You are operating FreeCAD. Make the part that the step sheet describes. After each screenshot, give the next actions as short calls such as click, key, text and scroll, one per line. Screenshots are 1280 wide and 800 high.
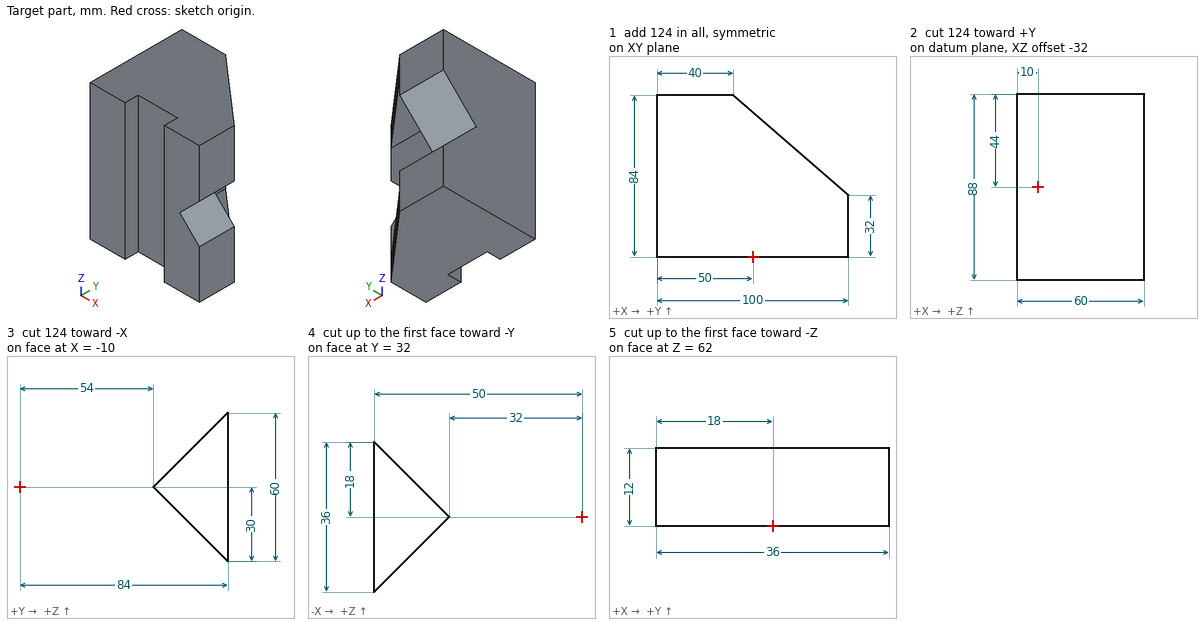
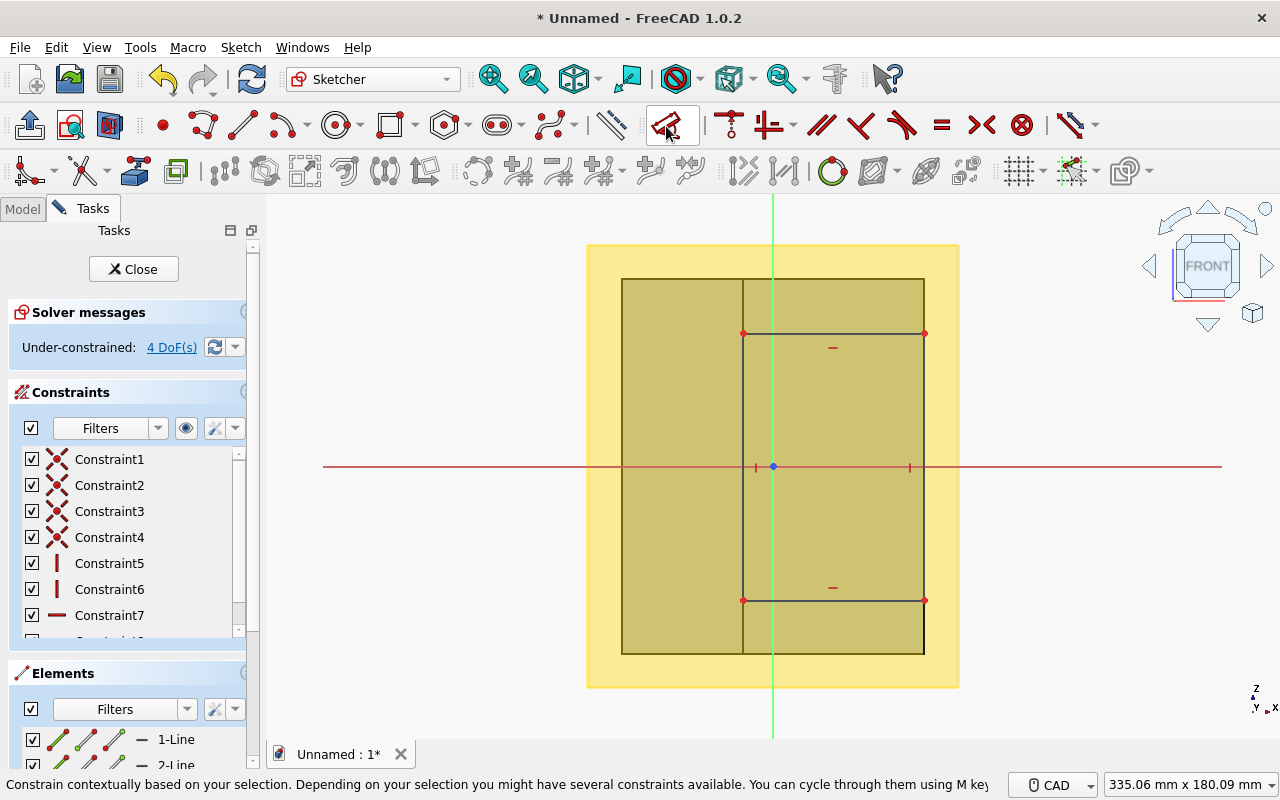
click(743, 414)
click(709, 406)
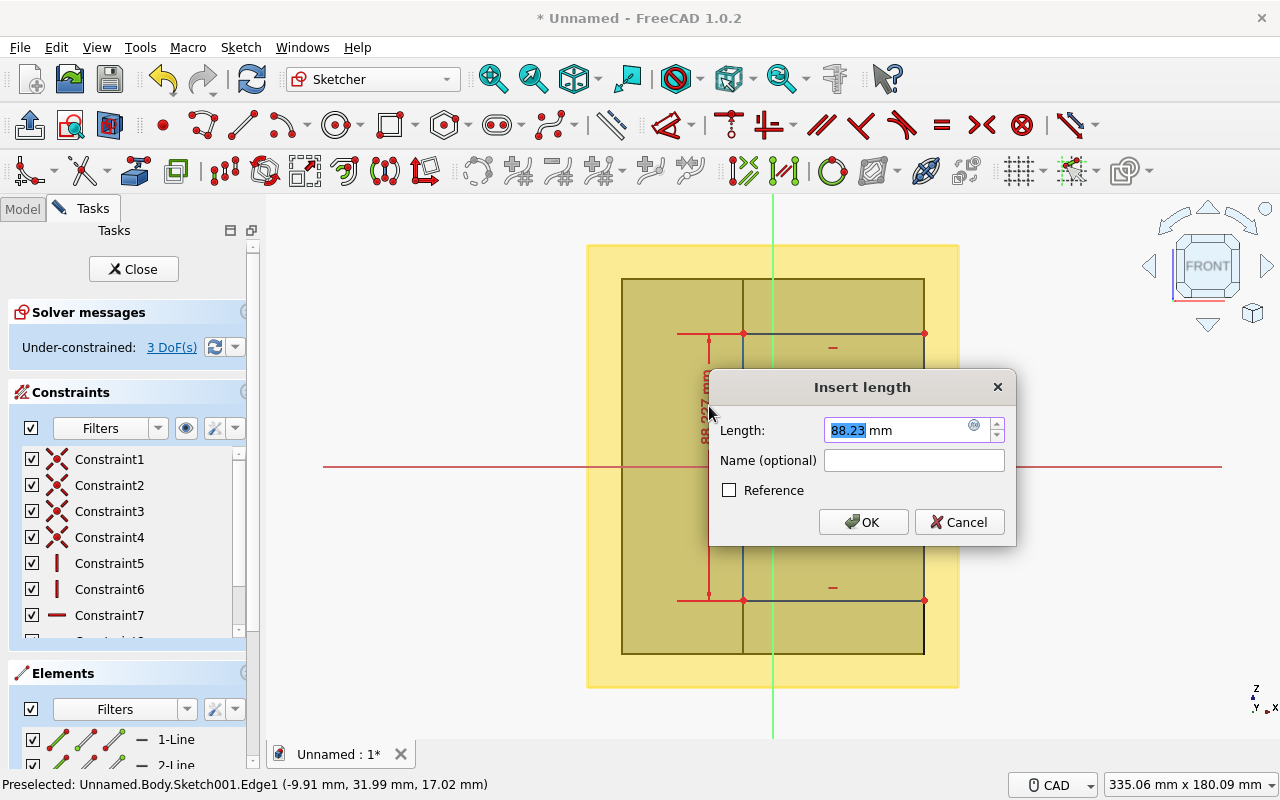
text(88)
key(Return)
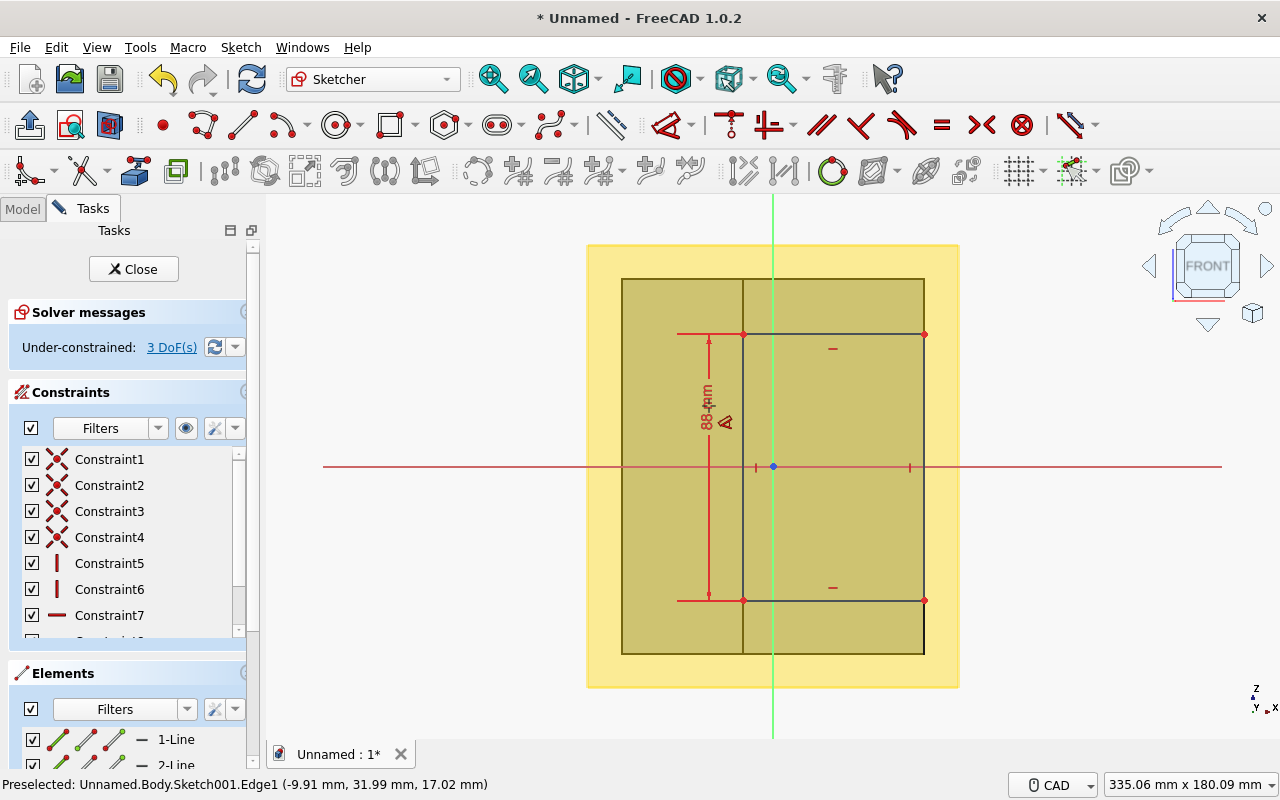
click(797, 601)
click(833, 635)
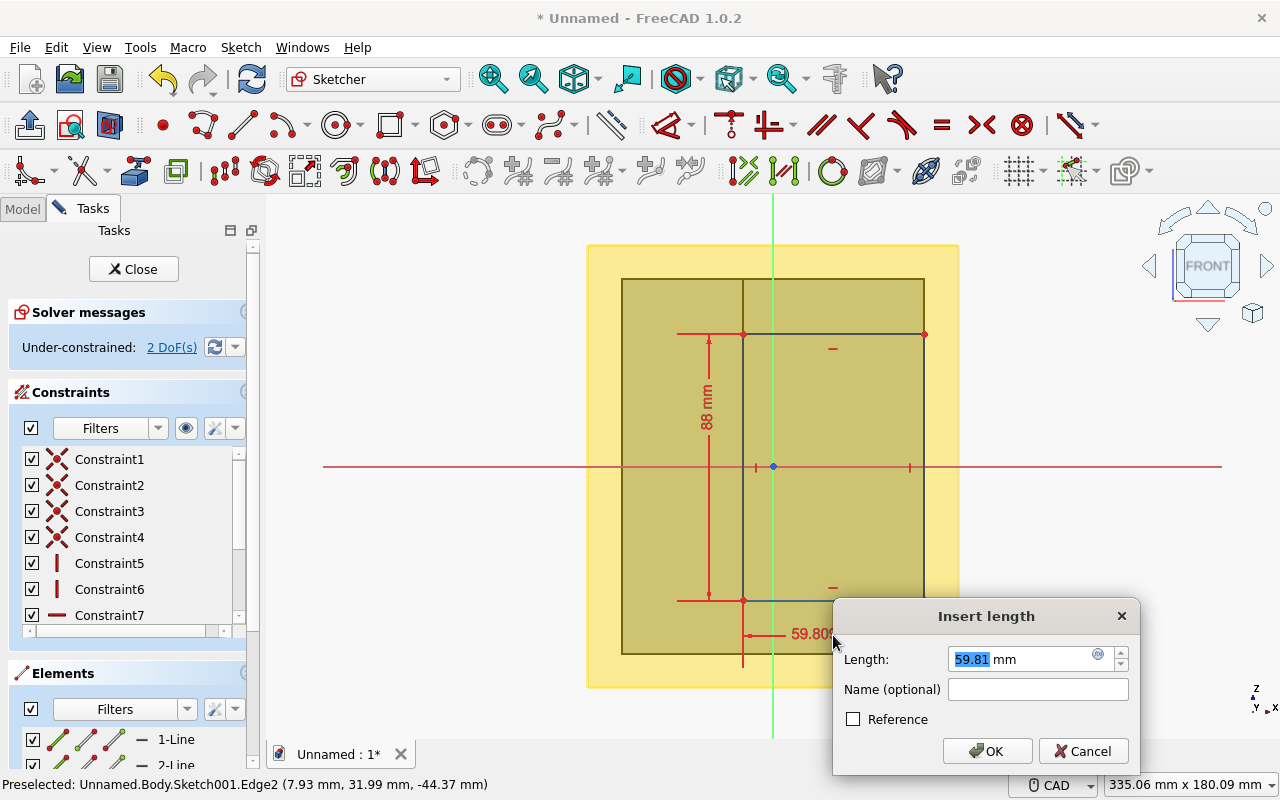
text(60)
key(Return)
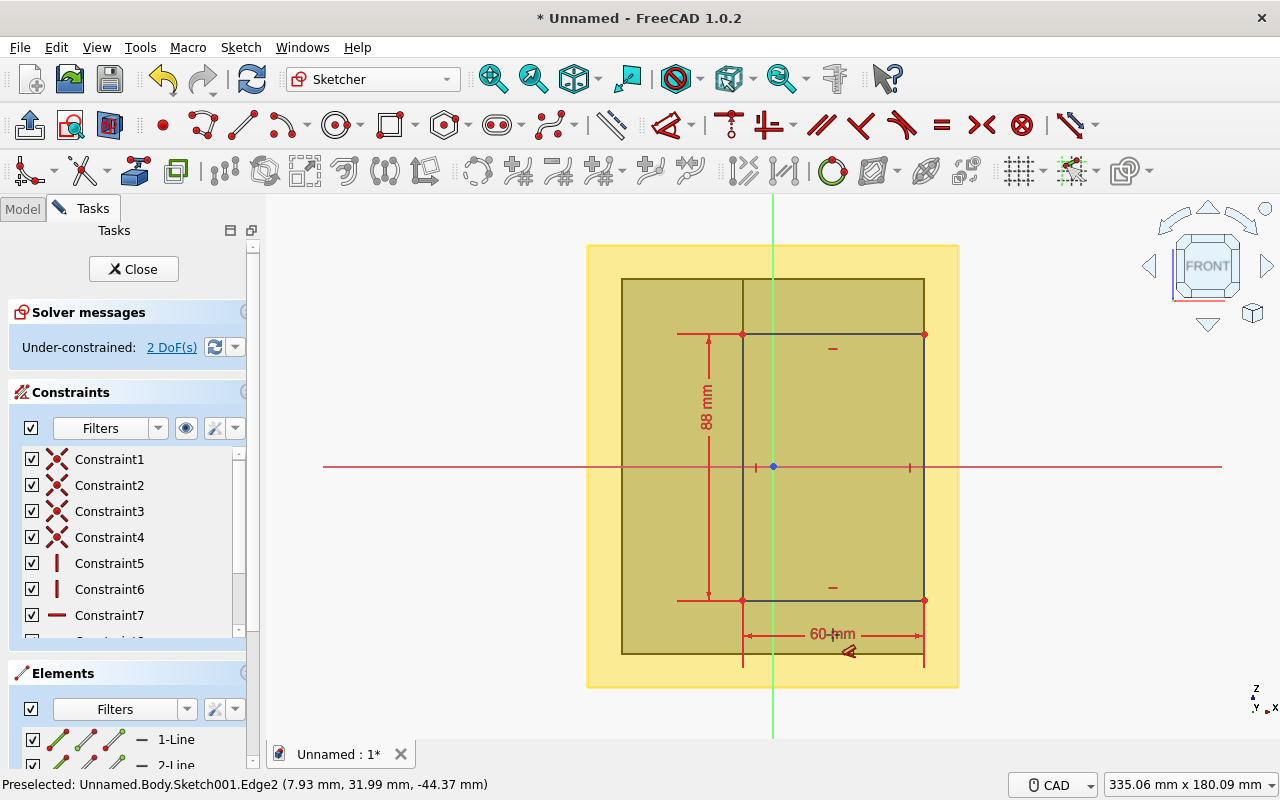
scroll(743, 334, up, 2)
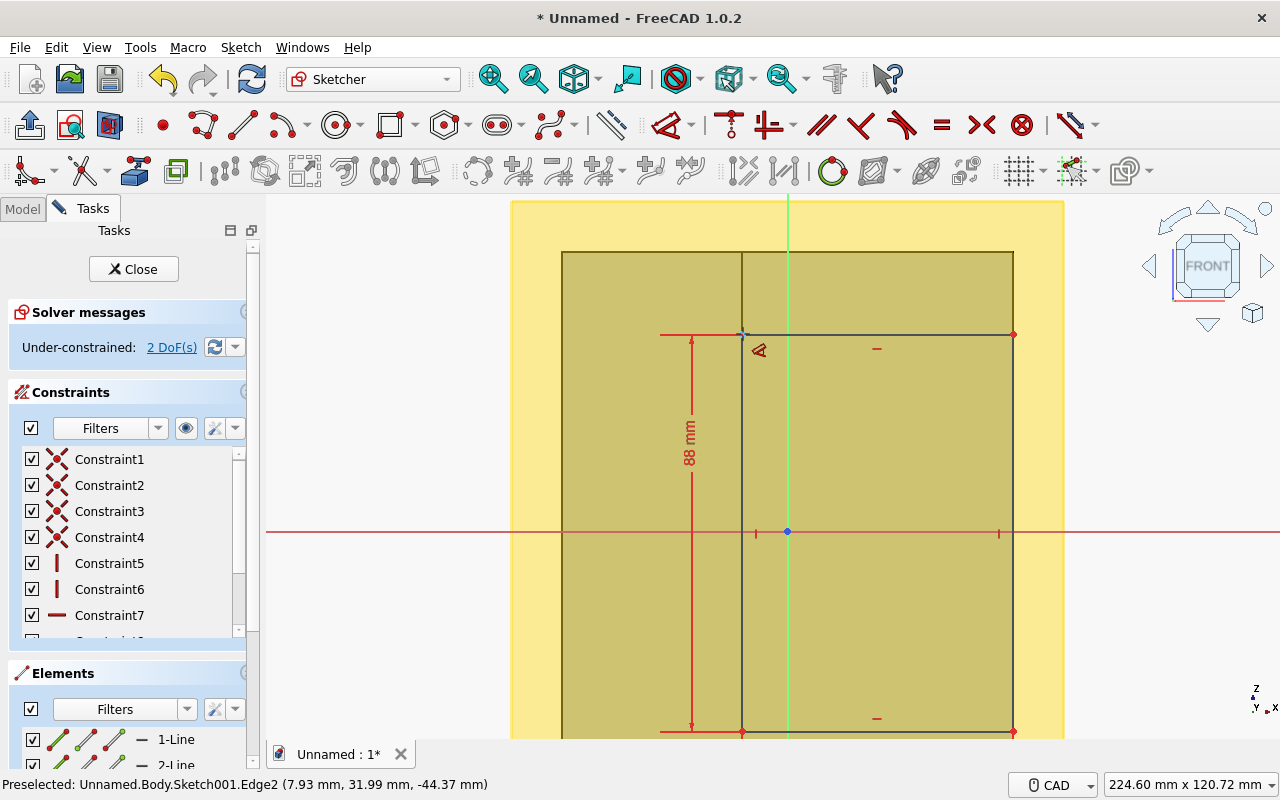
click(742, 335)
click(765, 301)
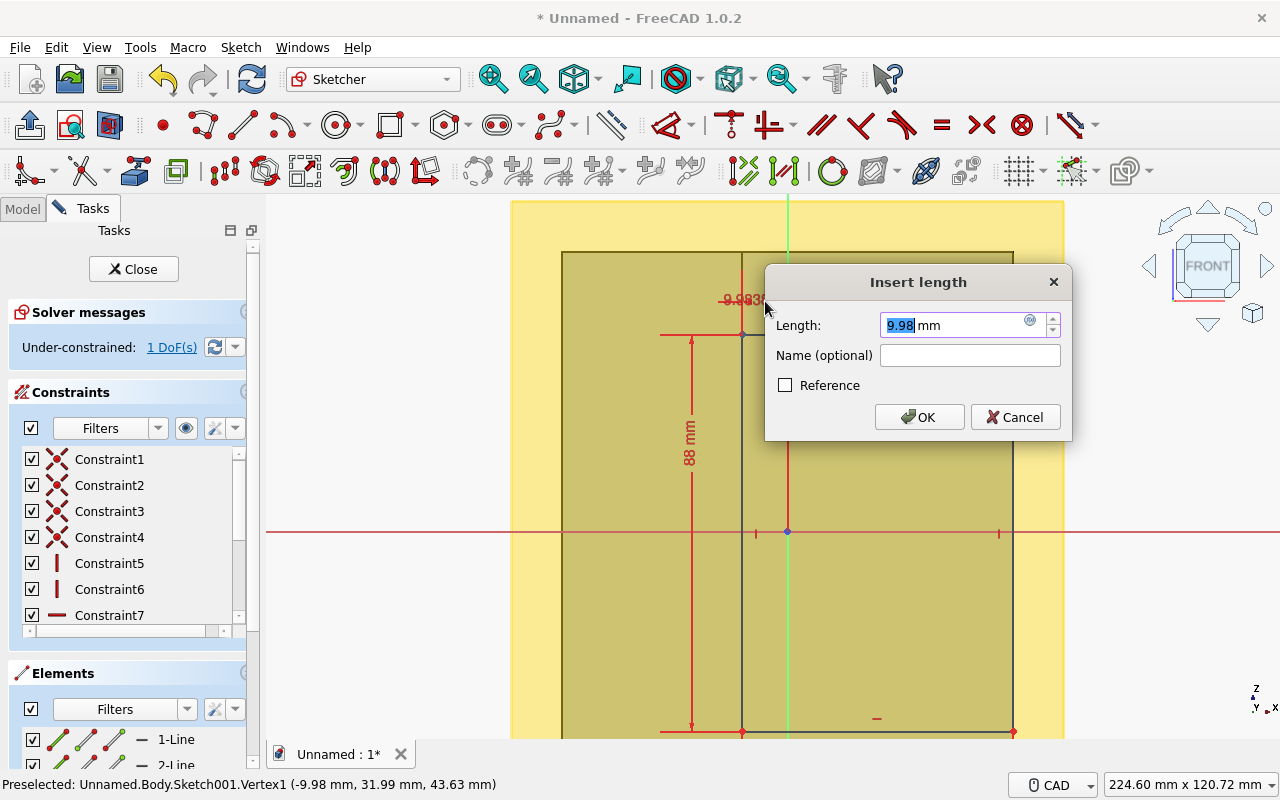
text(10)
key(Return)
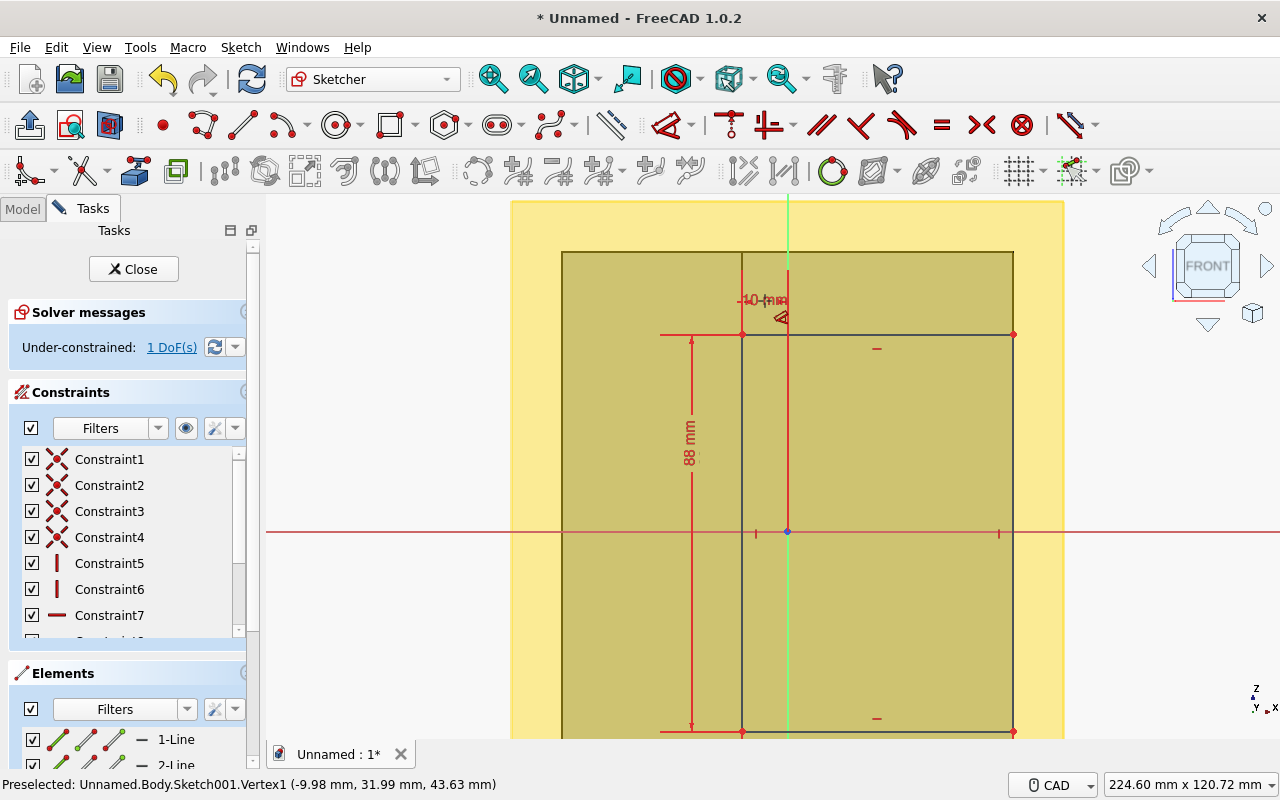
click(742, 335)
click(708, 388)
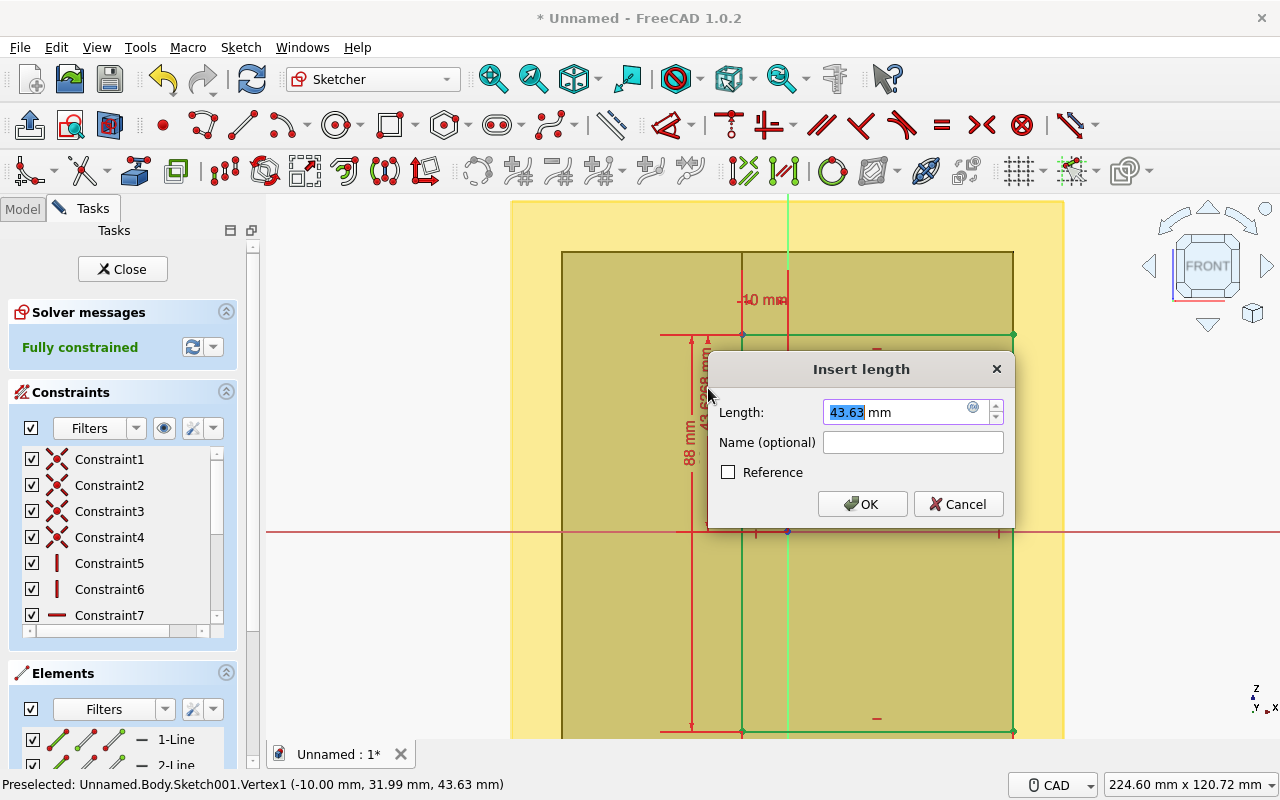
text(44)
key(Return)
key(Escape)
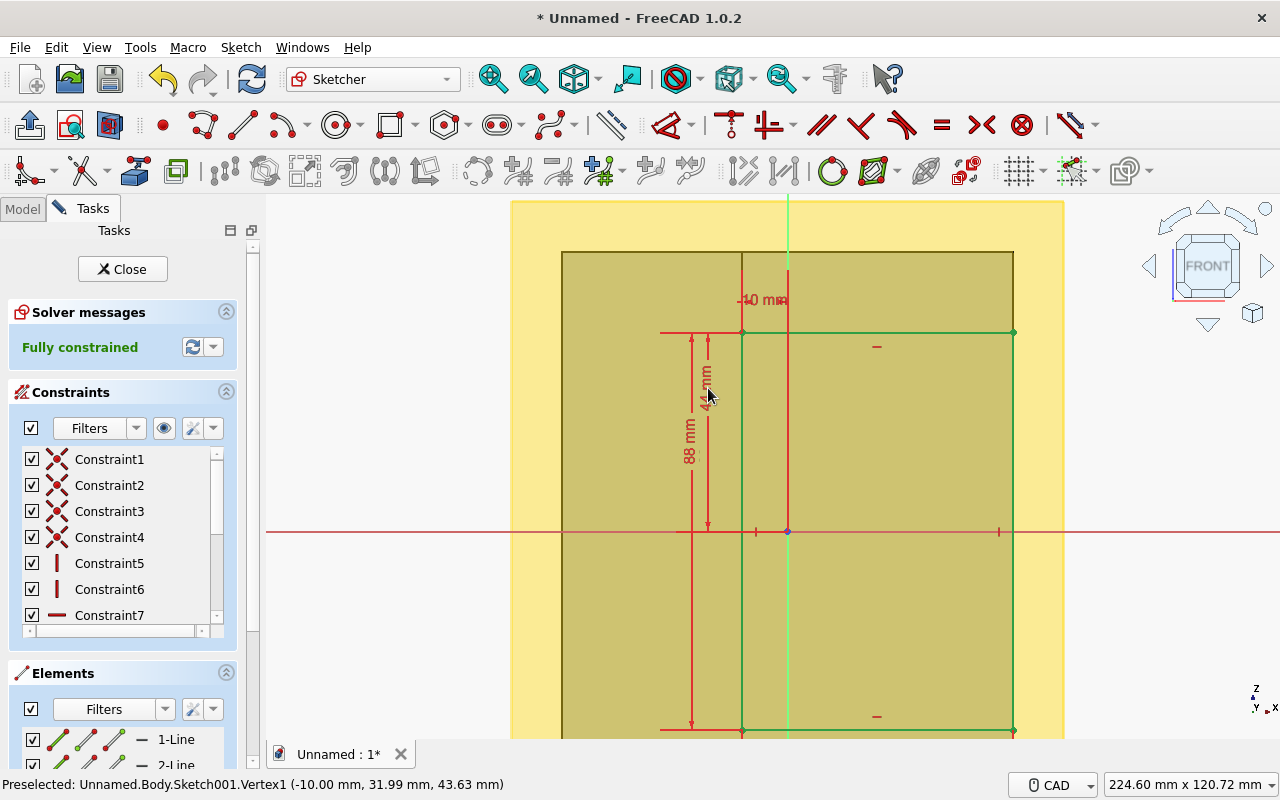
click(123, 269)